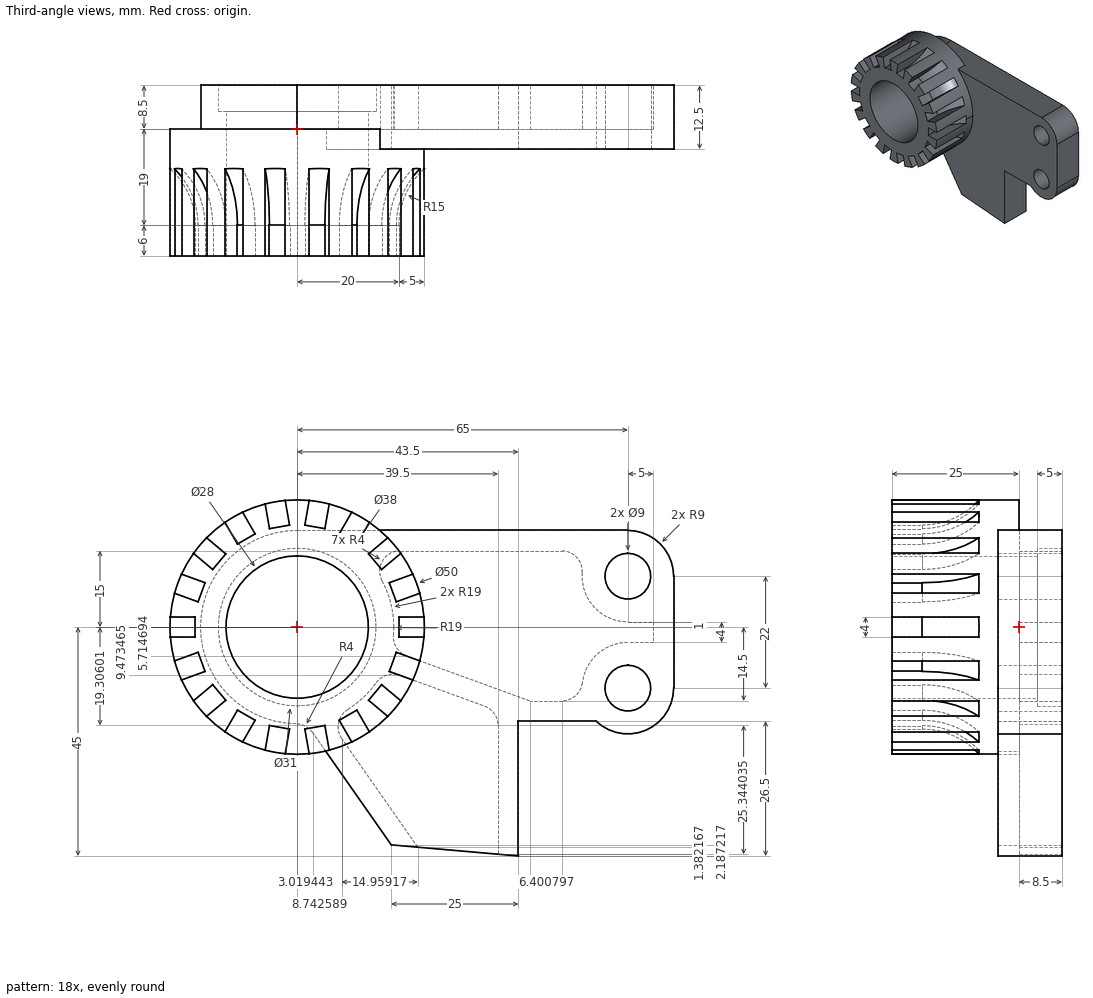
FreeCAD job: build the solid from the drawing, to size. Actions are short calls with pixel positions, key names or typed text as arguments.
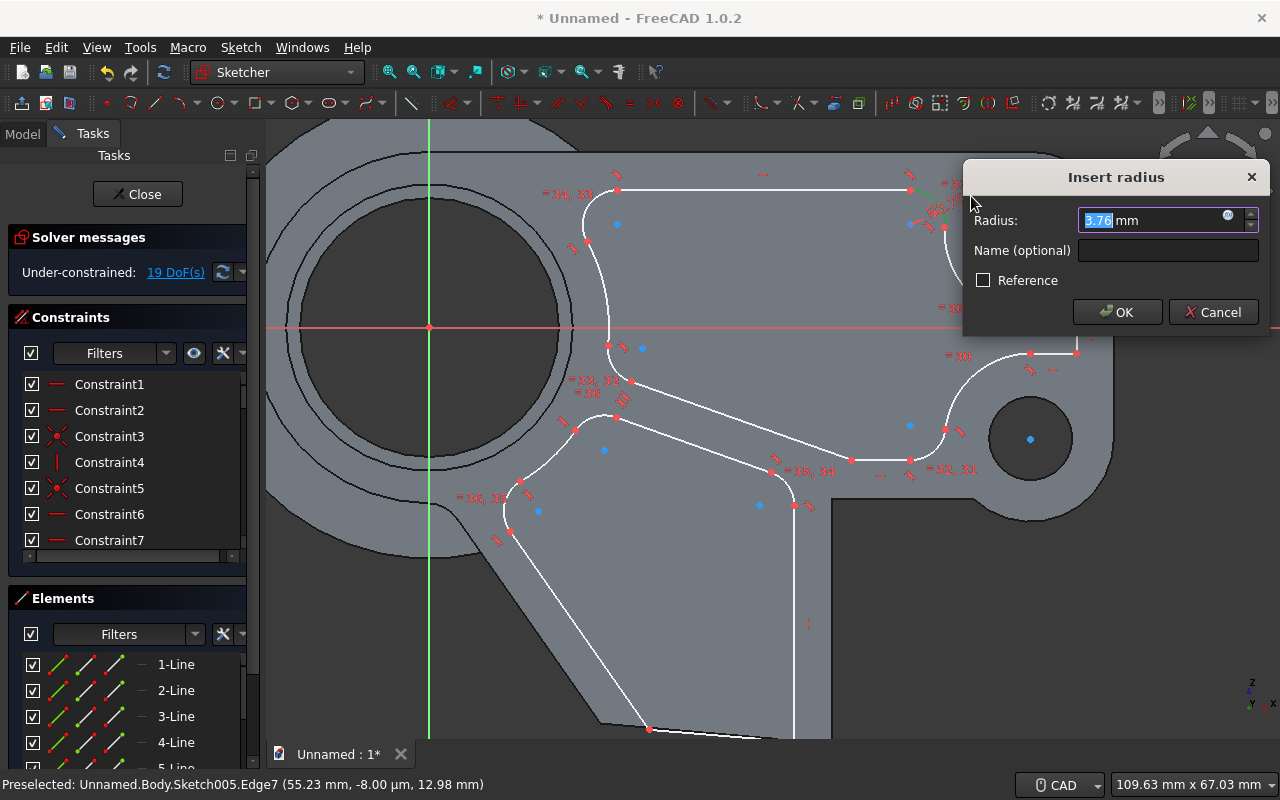
text(4)
key(Return)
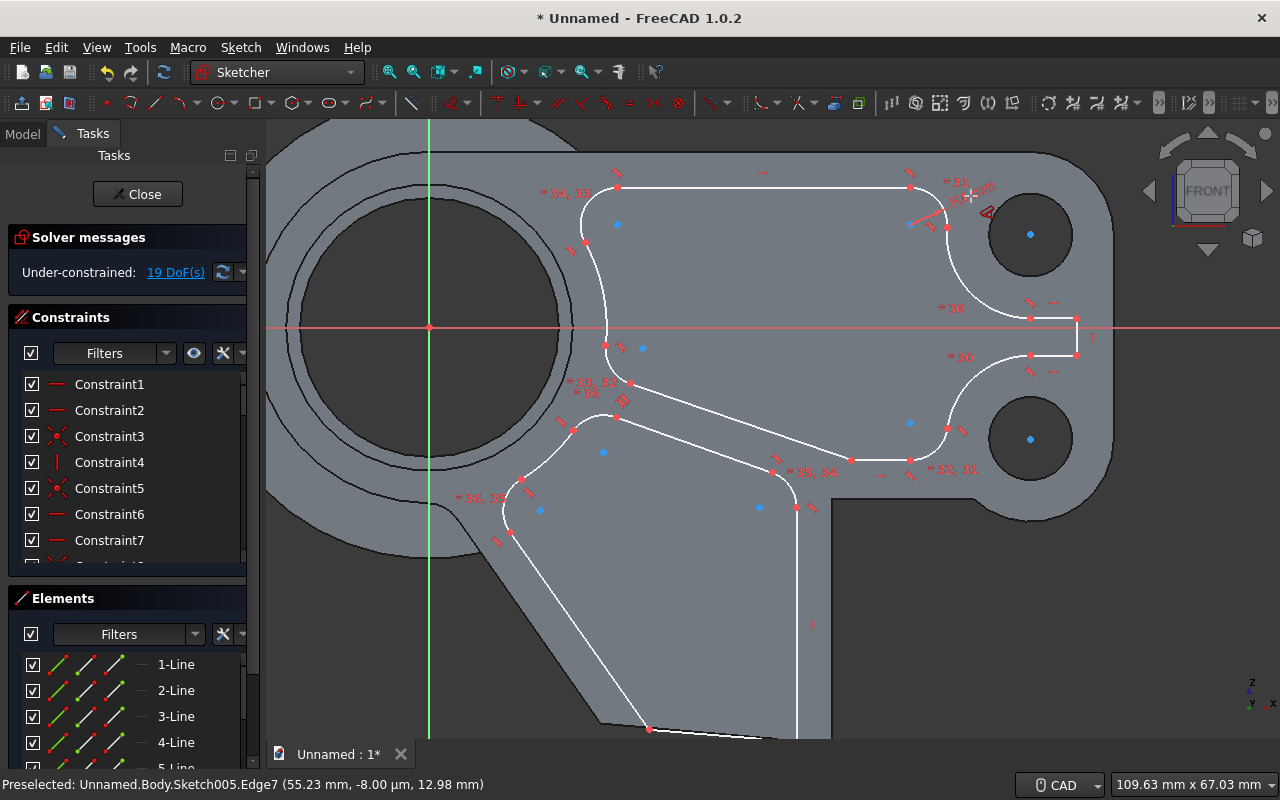
click(954, 268)
click(925, 281)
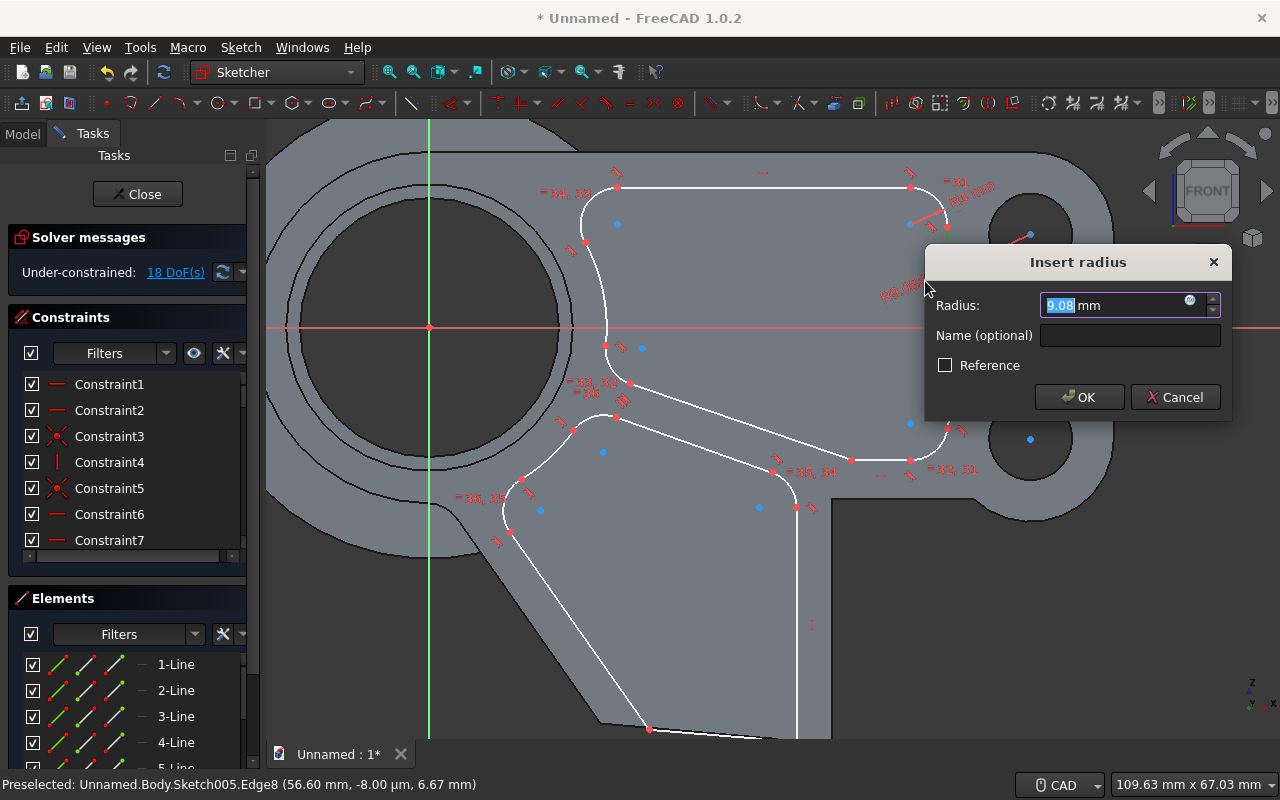
text(9)
key(Return)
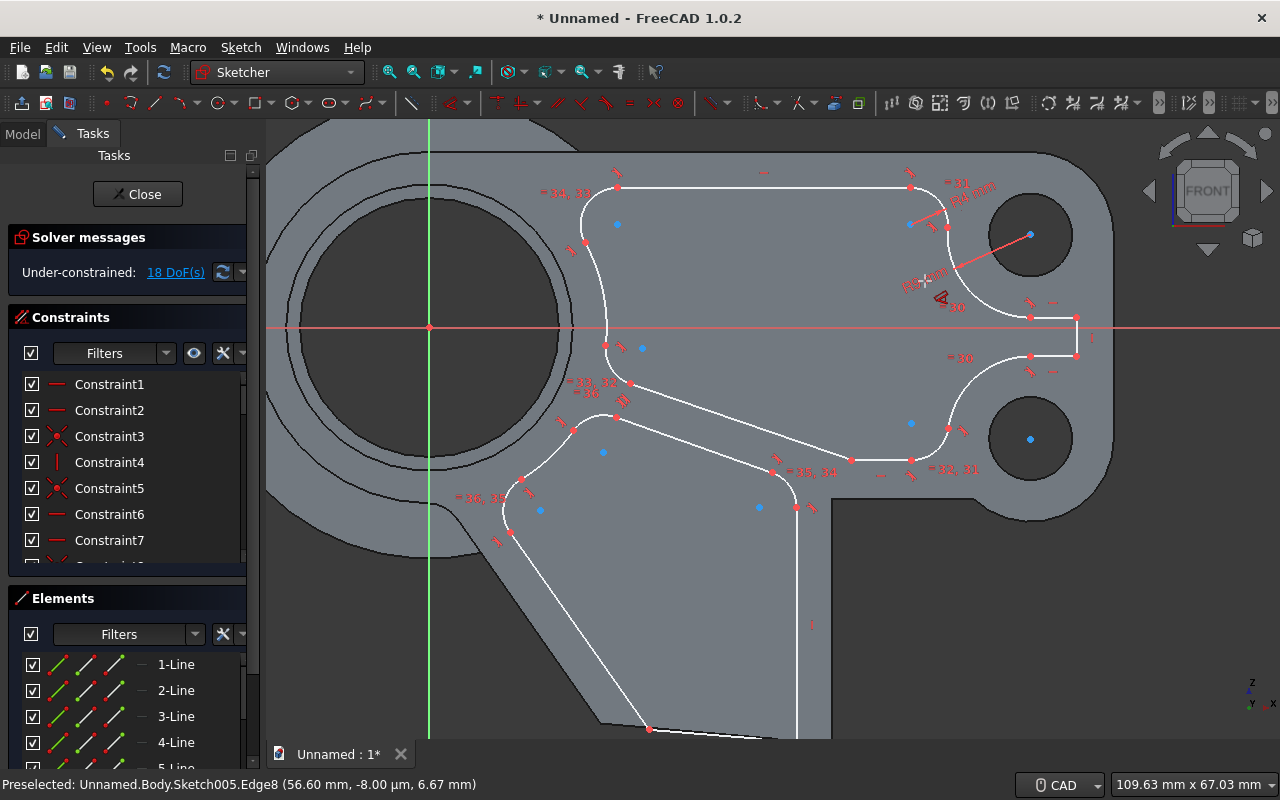
click(606, 313)
click(638, 310)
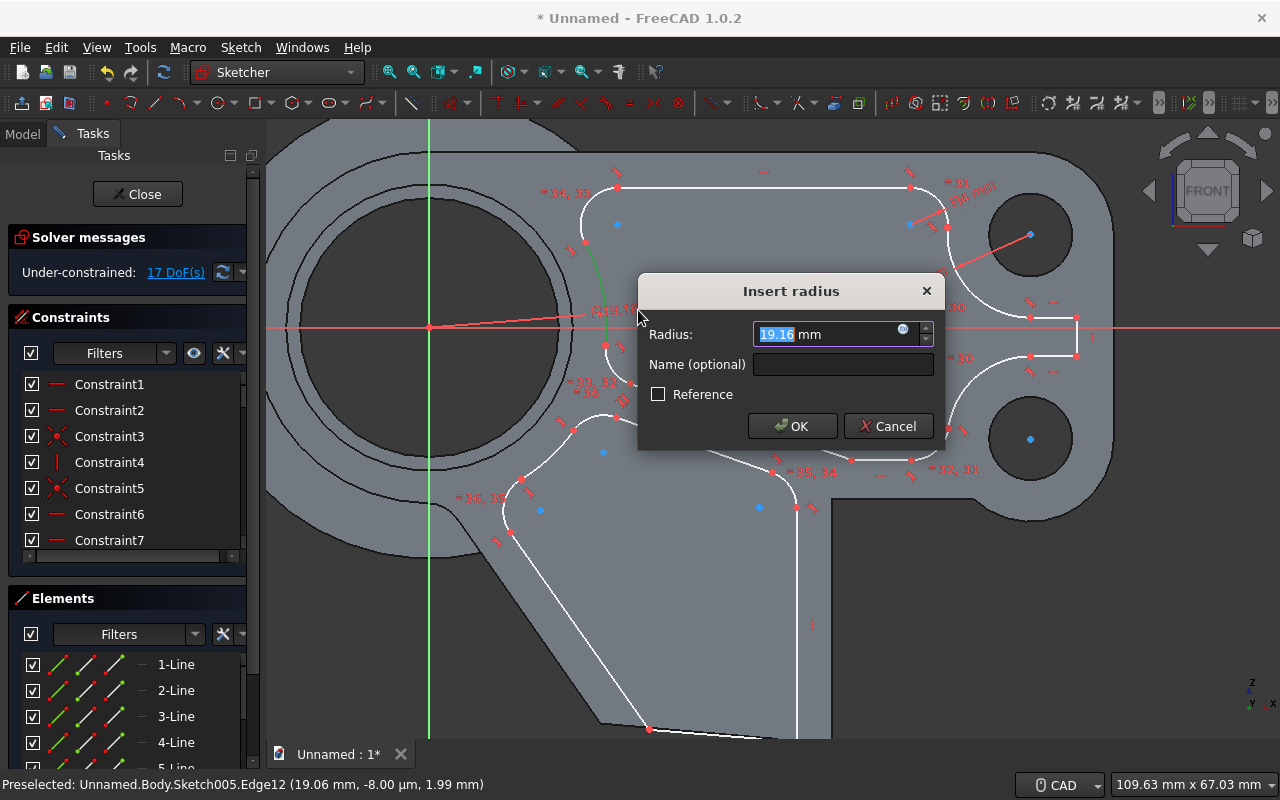
text(19)
key(Return)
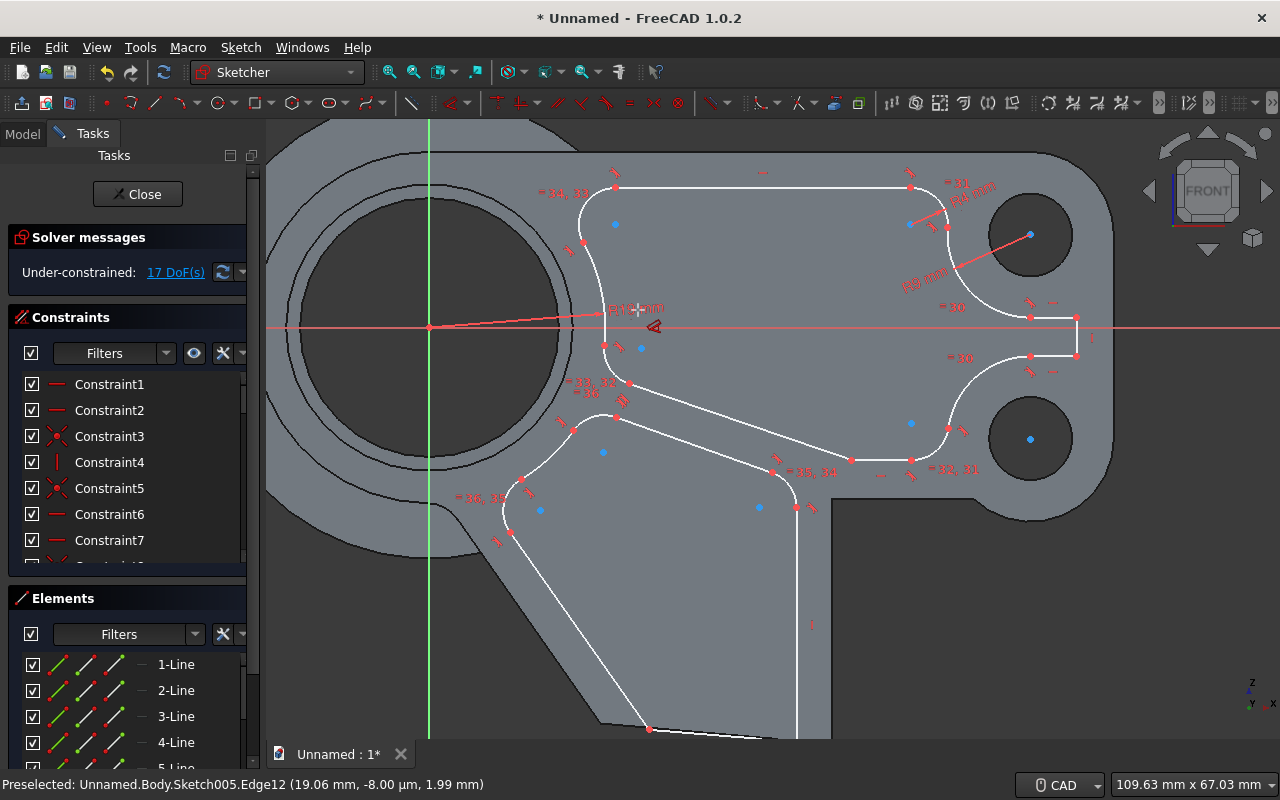
click(539, 467)
click(559, 492)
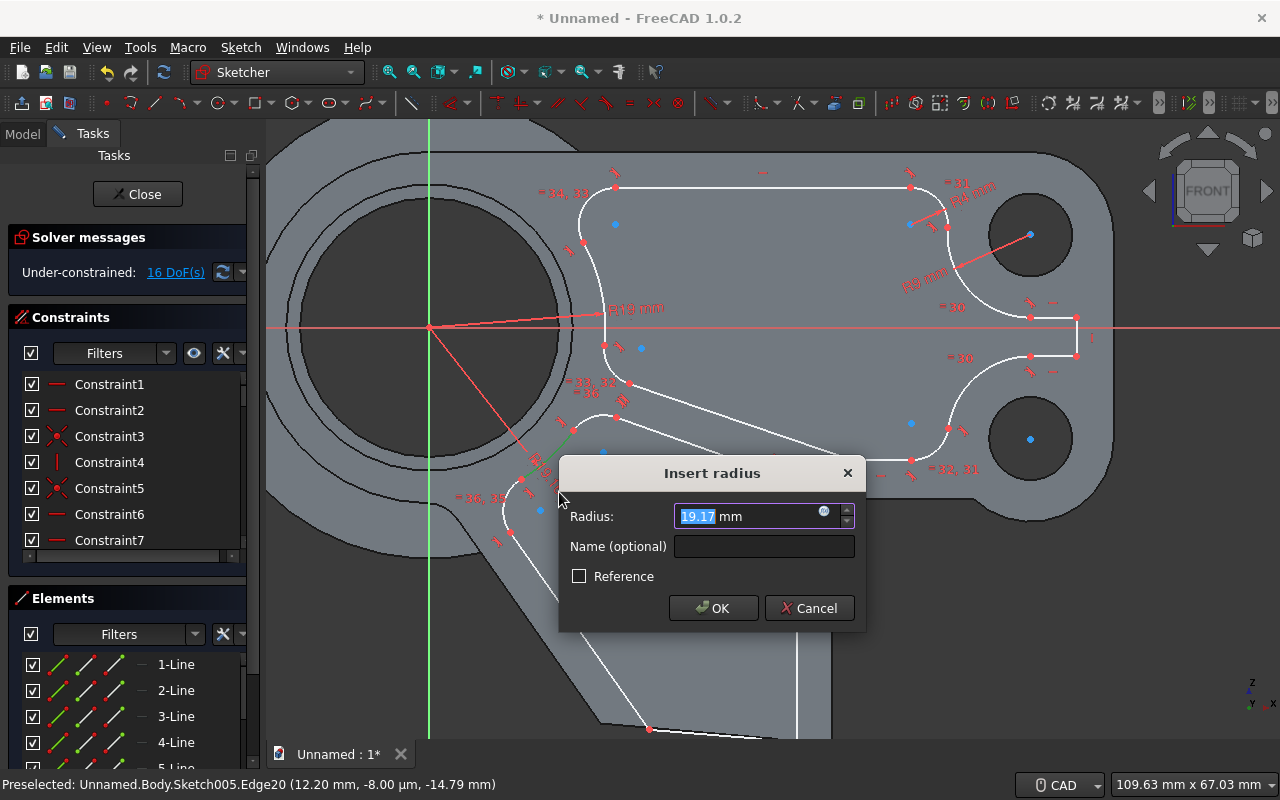
text(19)
key(Return)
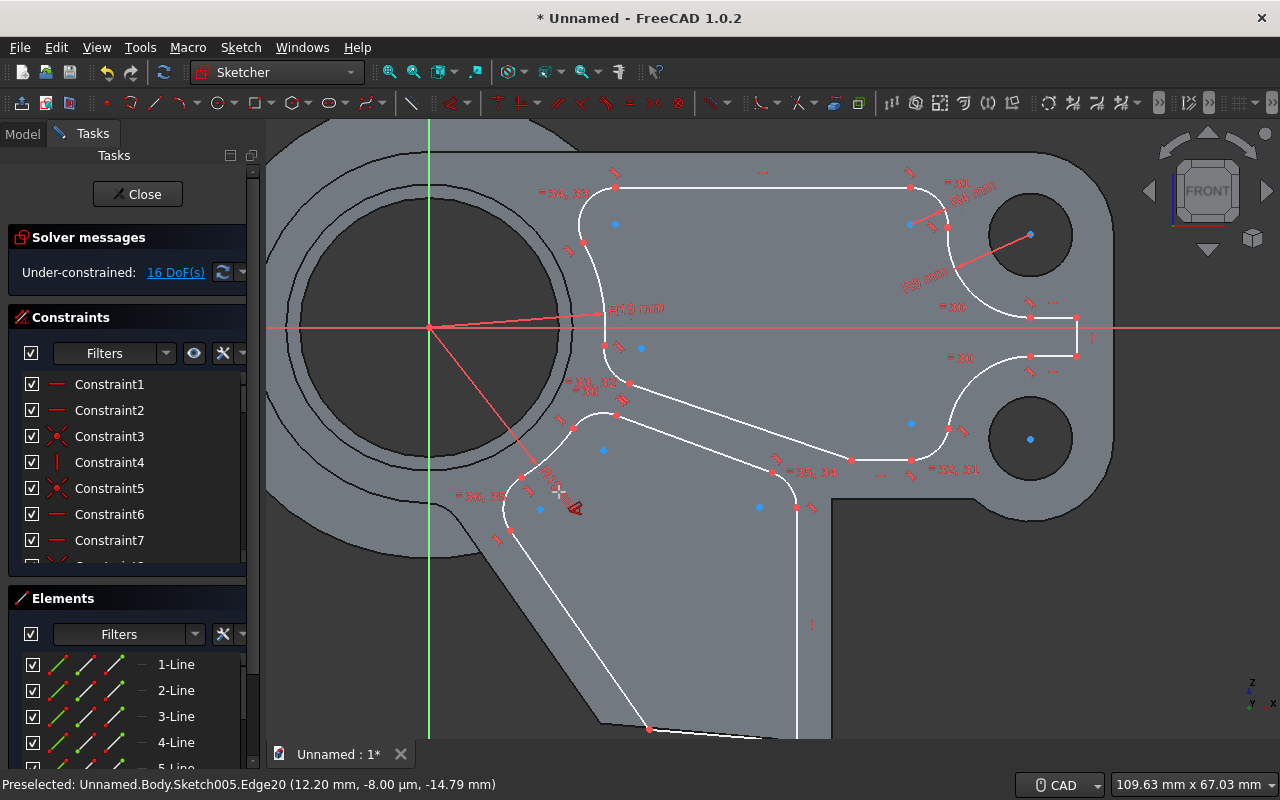
scroll(1045, 318, up, 2)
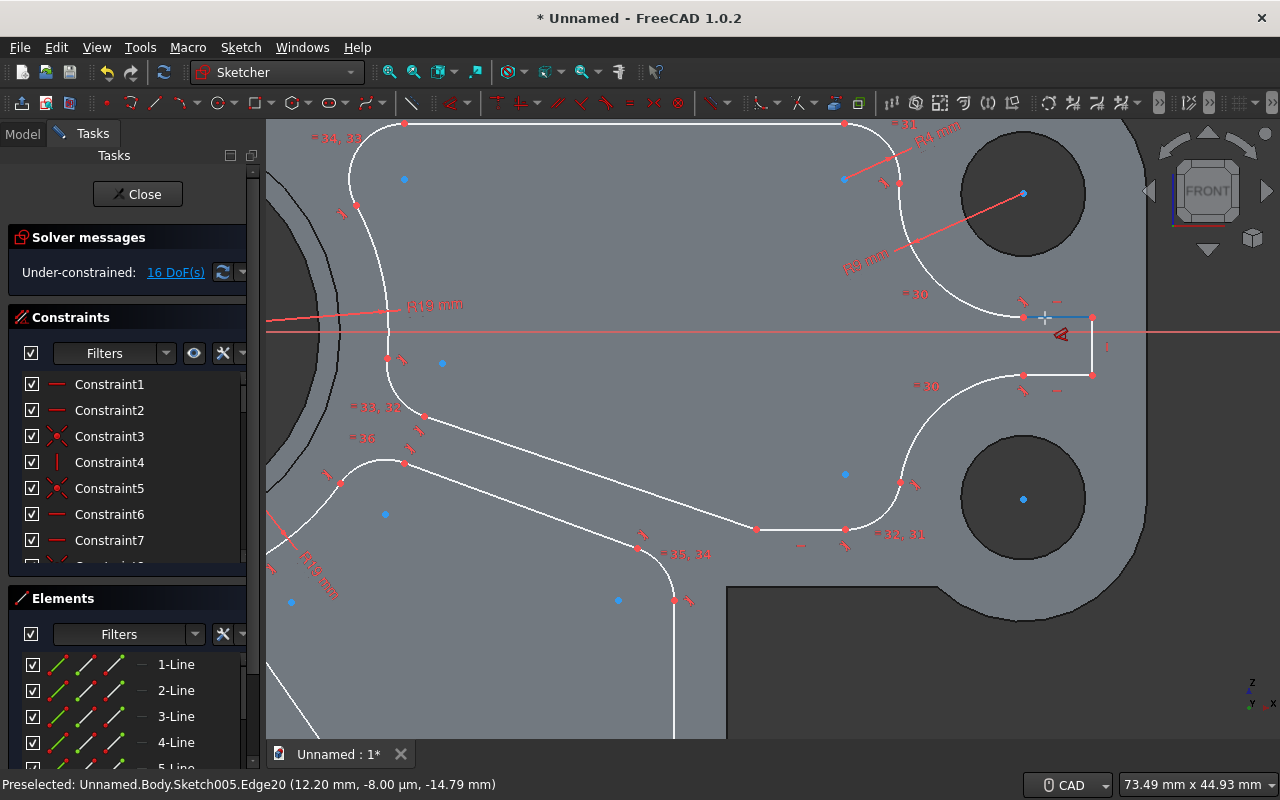
click(1044, 317)
click(1058, 283)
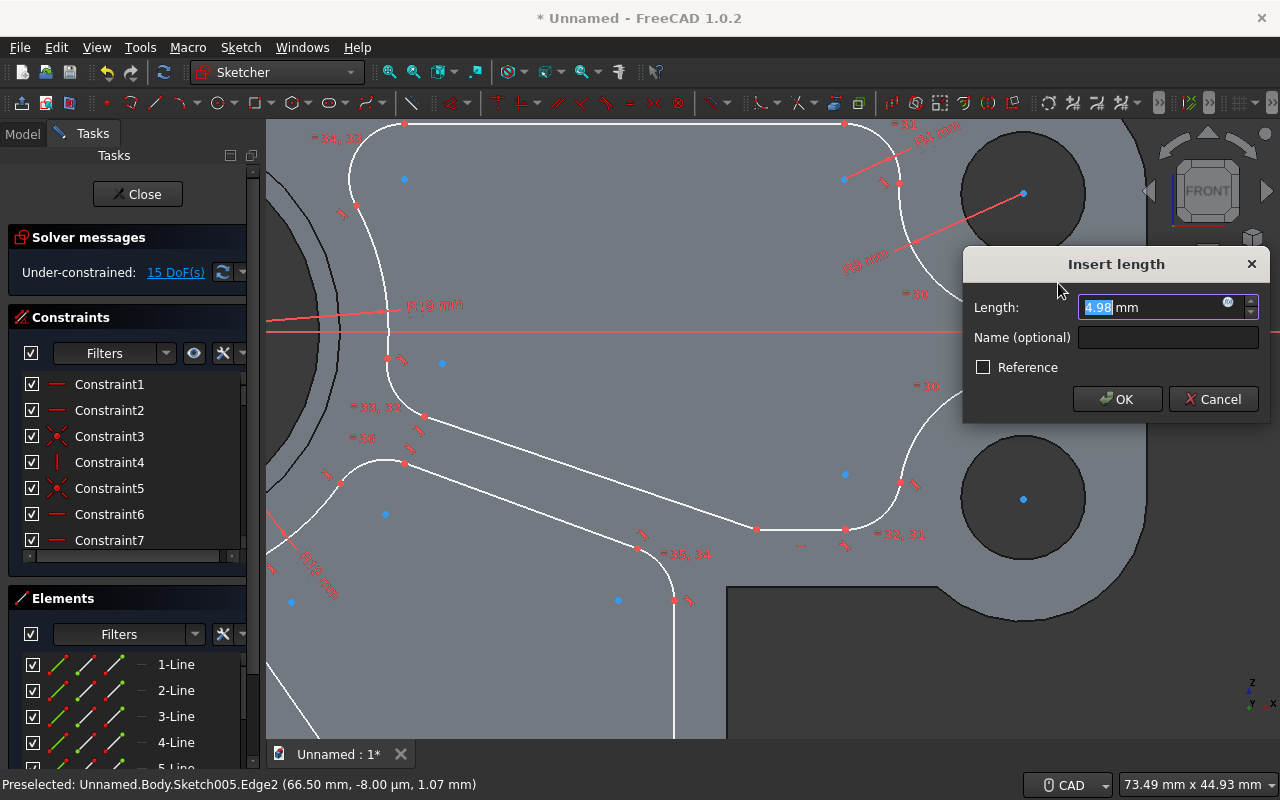
text(5)
key(Return)